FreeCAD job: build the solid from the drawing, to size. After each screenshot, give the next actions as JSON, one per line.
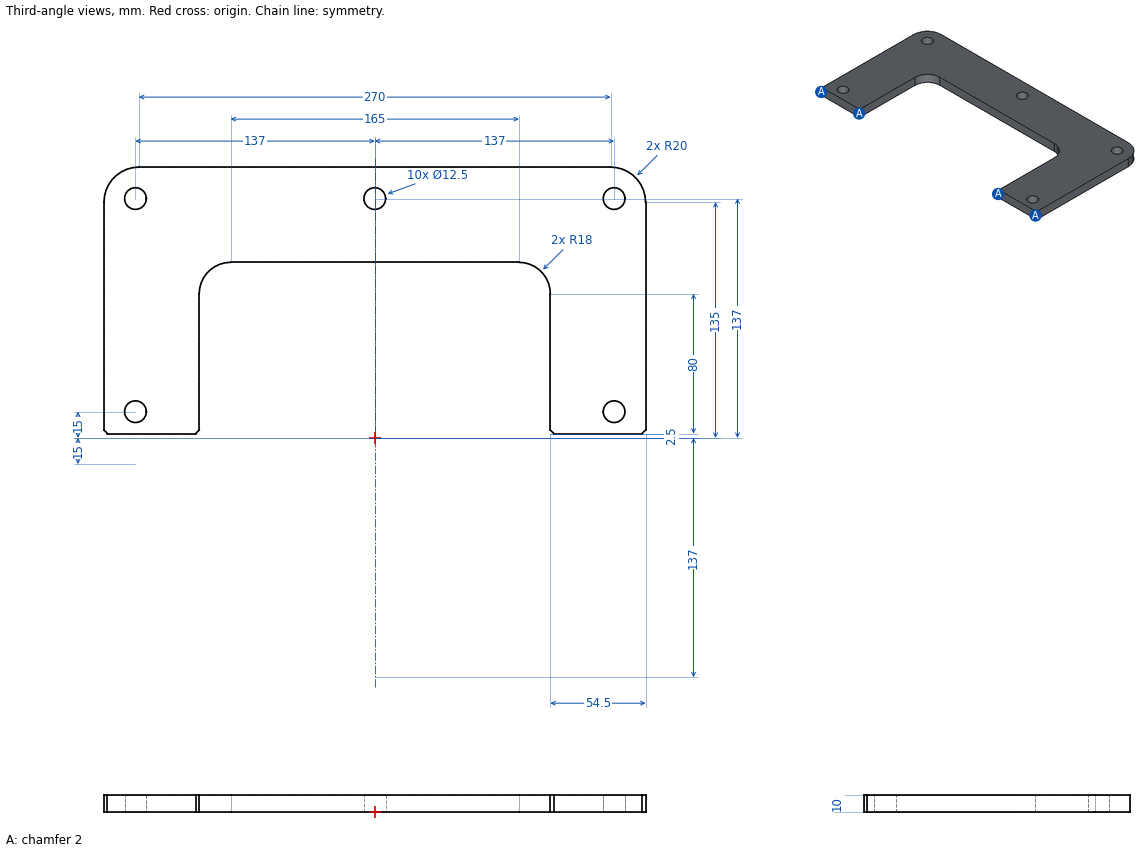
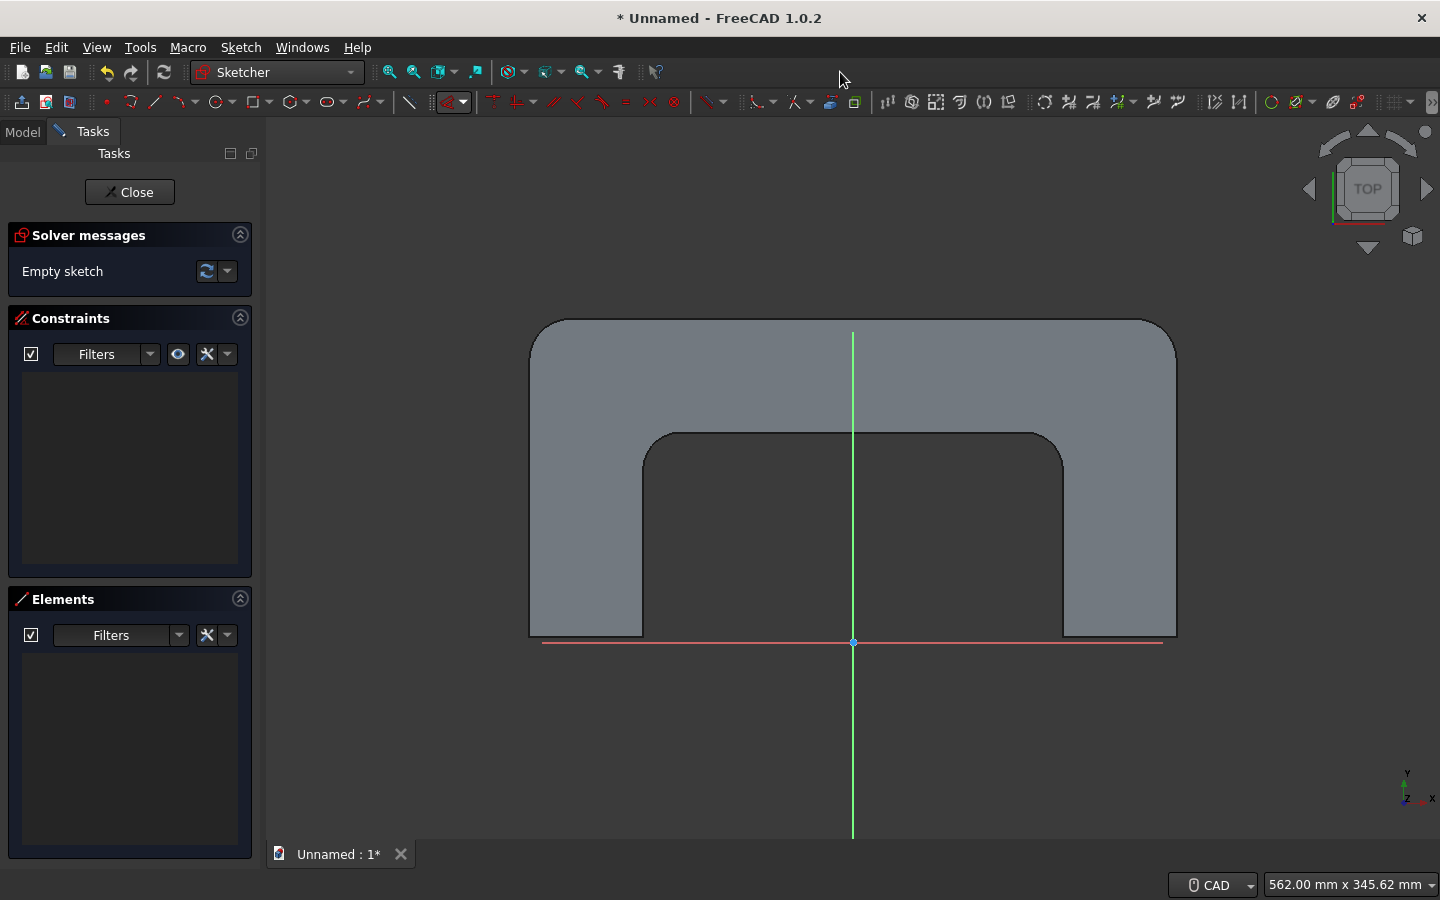
{"action": "scroll", "coordinate": [645, 145], "scroll_direction": "down", "scroll_amount": 2}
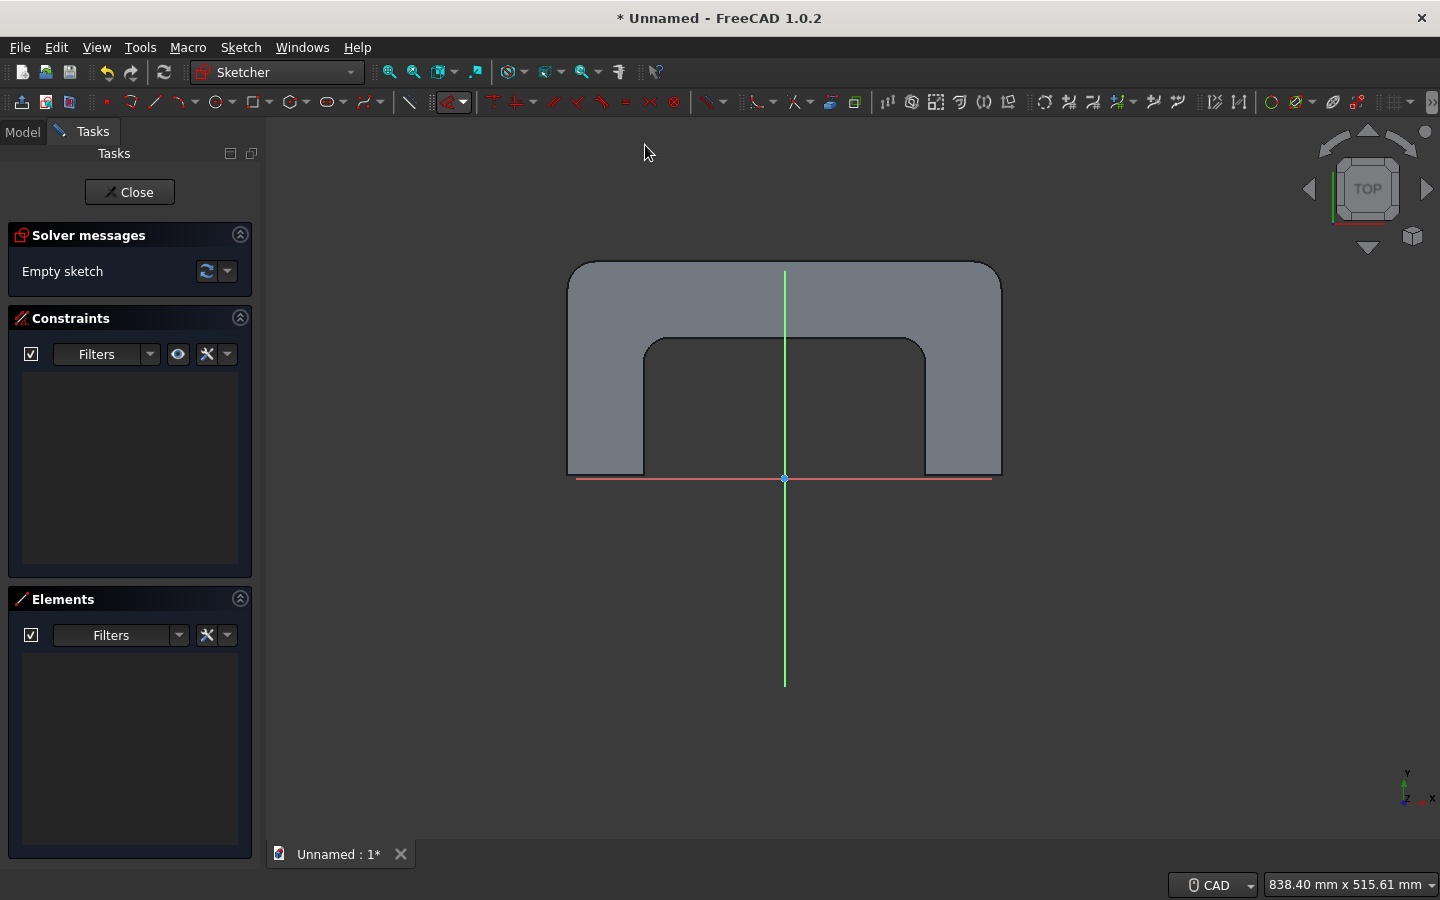
{"action": "key", "text": "g c"}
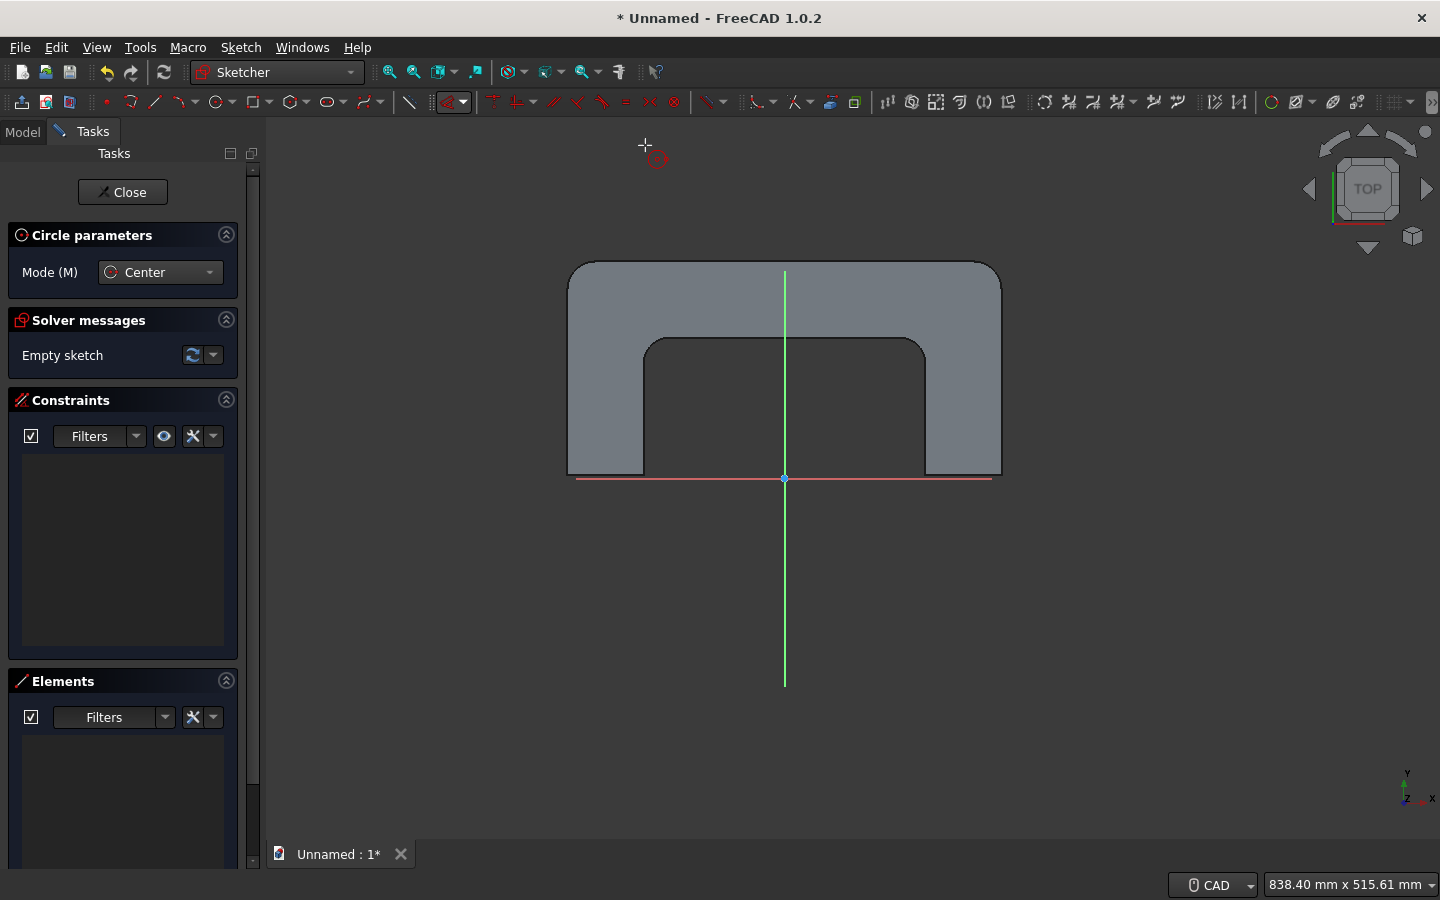
{"action": "scroll", "coordinate": [785, 287], "scroll_direction": "up", "scroll_amount": 5}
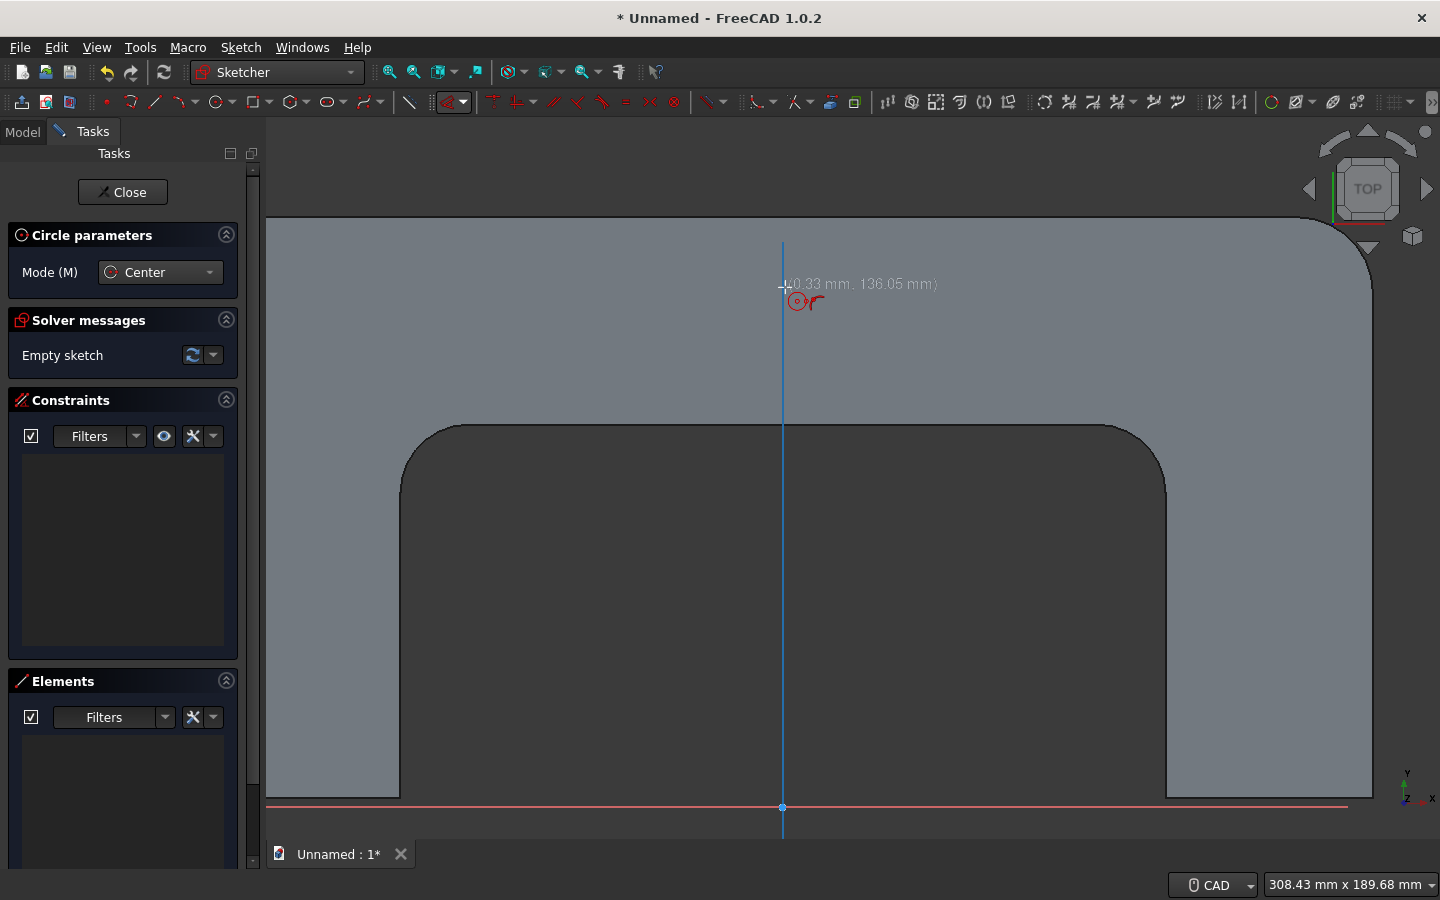
{"action": "left_click", "coordinate": [783, 286]}
{"action": "mouse_move", "coordinate": [800, 269]}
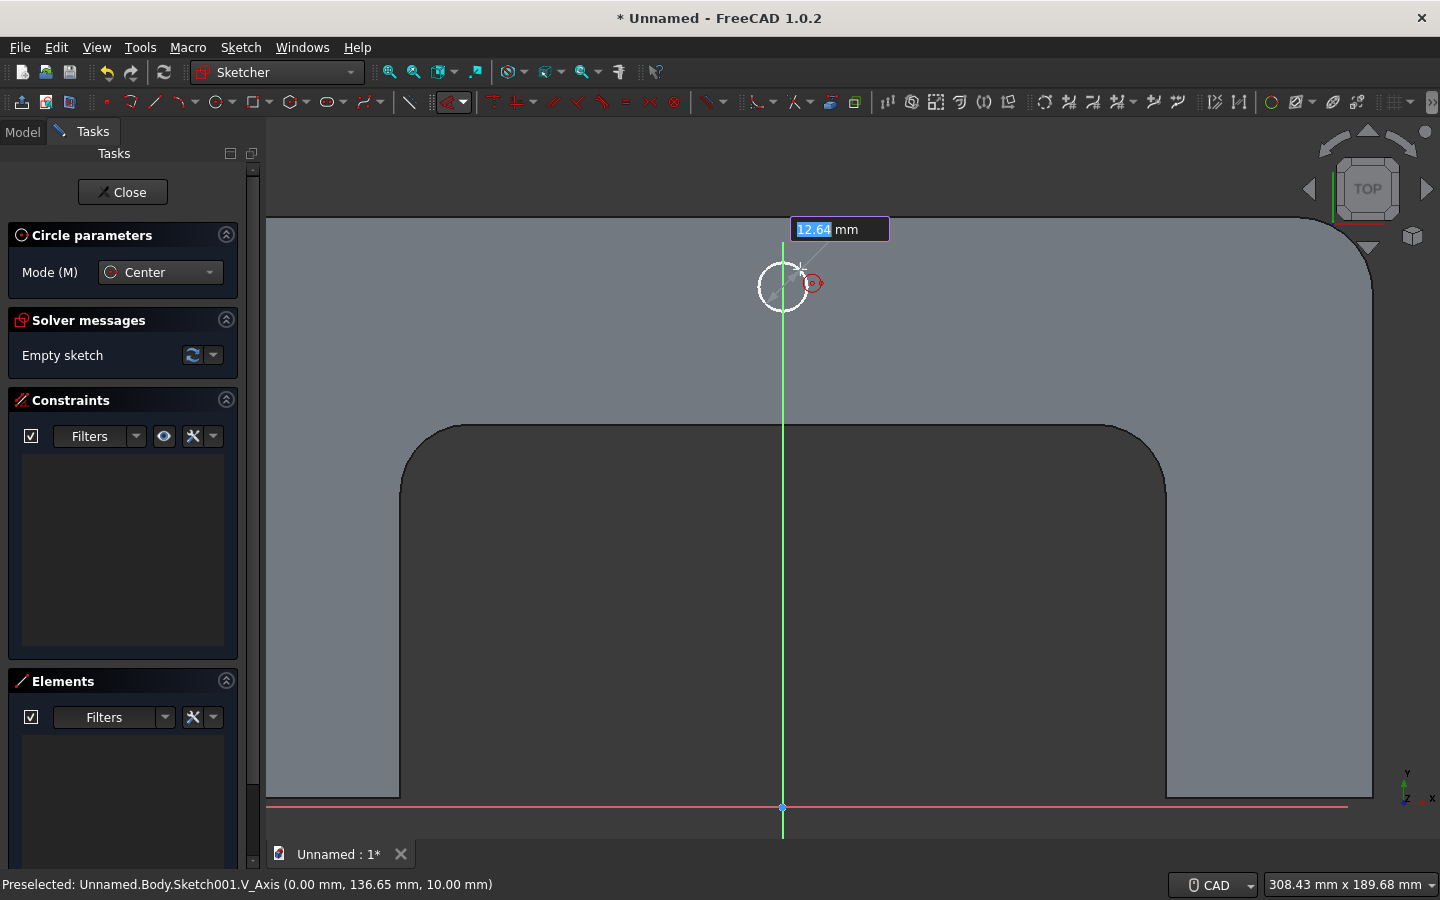
{"action": "type", "text": "12.5"}
{"action": "key", "text": "Return"}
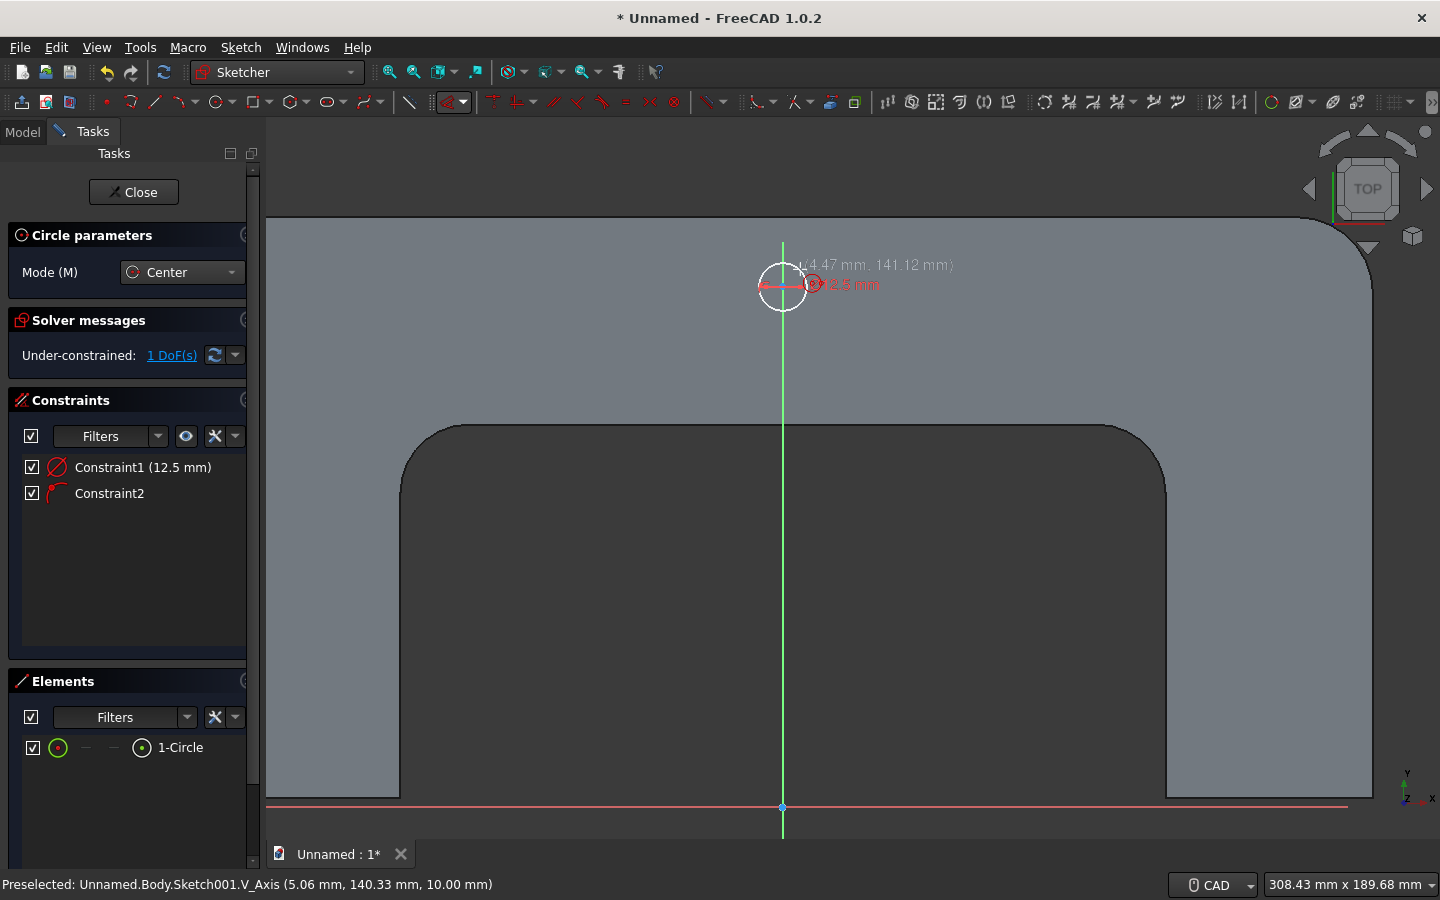
{"action": "scroll", "coordinate": [786, 209], "scroll_direction": "down", "scroll_amount": 4}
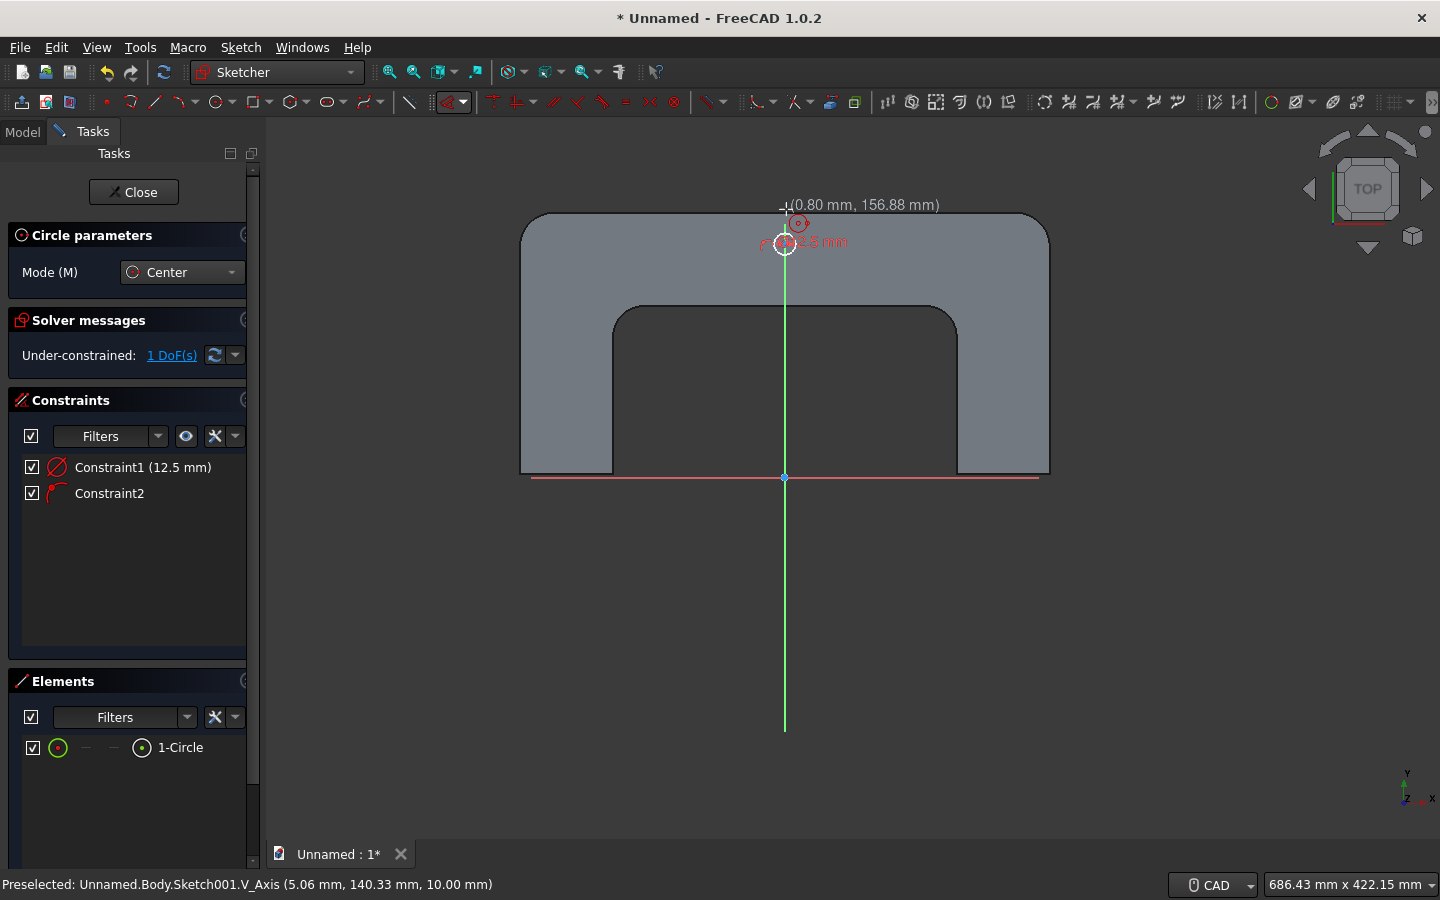
{"action": "scroll", "coordinate": [785, 712], "scroll_direction": "up", "scroll_amount": 4}